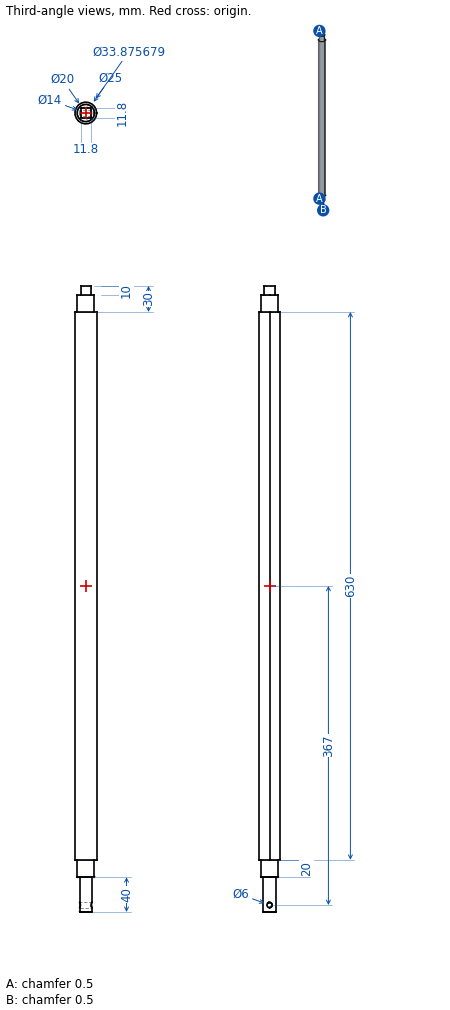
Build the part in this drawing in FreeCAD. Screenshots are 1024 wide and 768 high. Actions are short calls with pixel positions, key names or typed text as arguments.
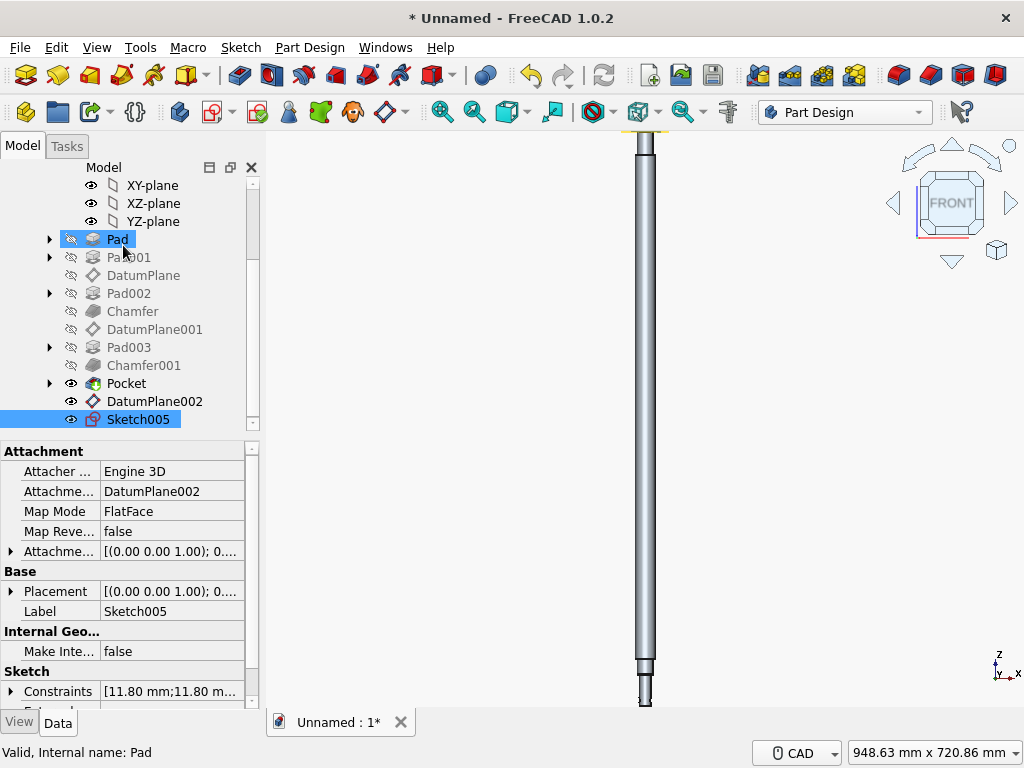
click(240, 76)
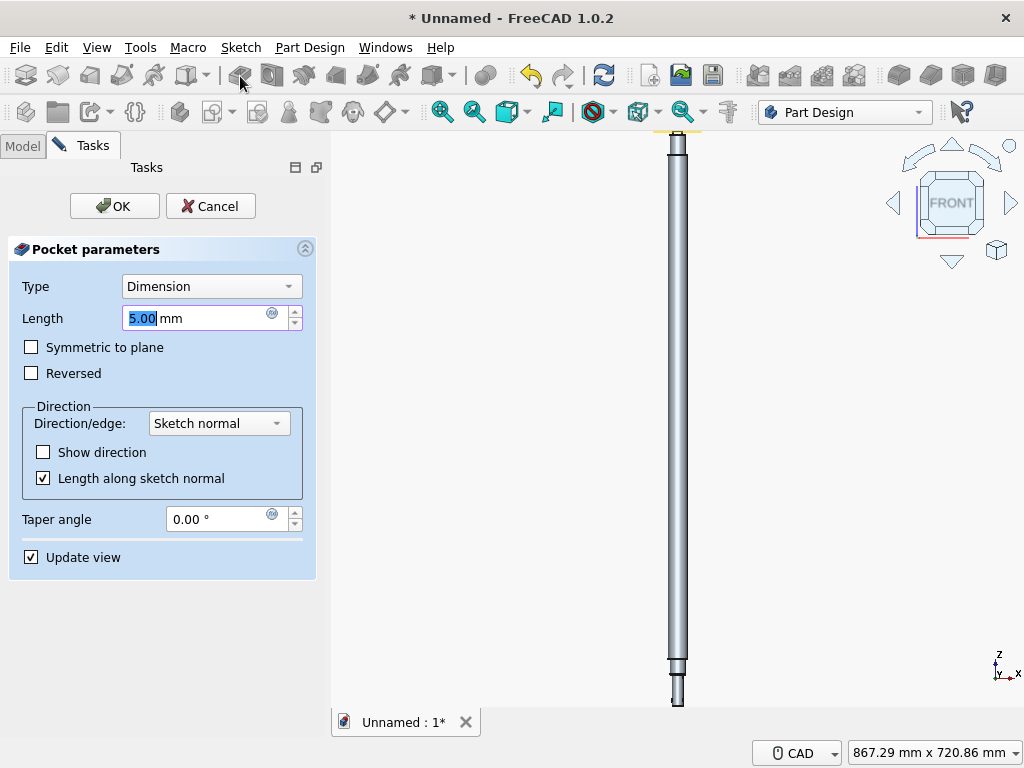
text(10)
key(Tab)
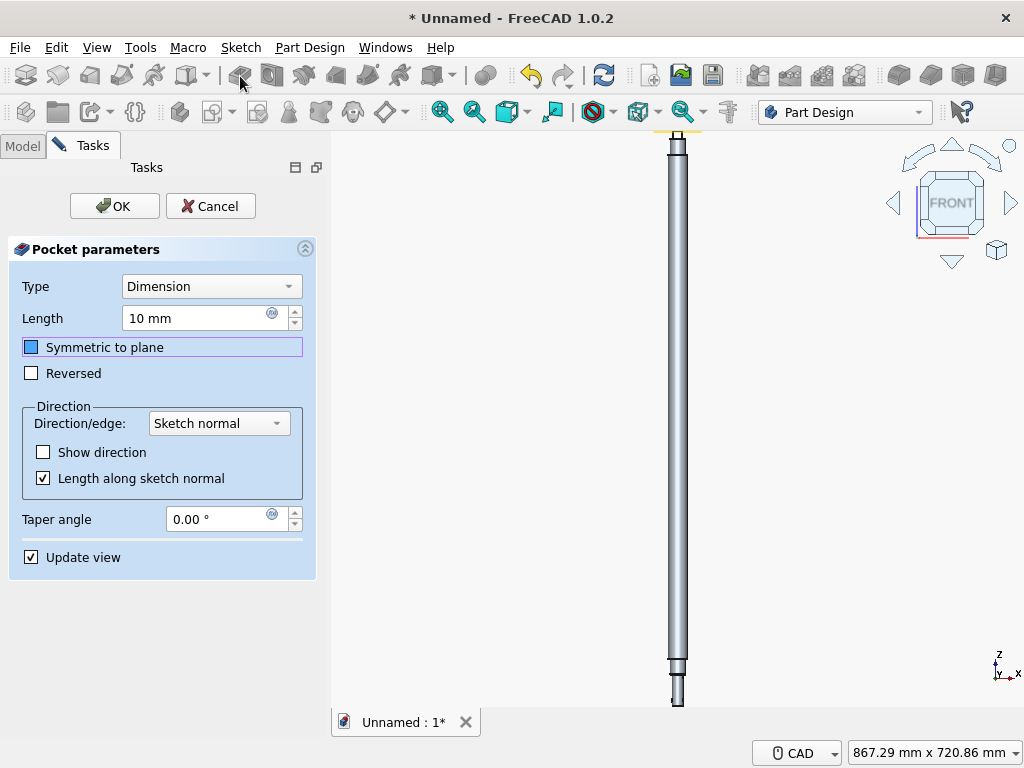
click(115, 206)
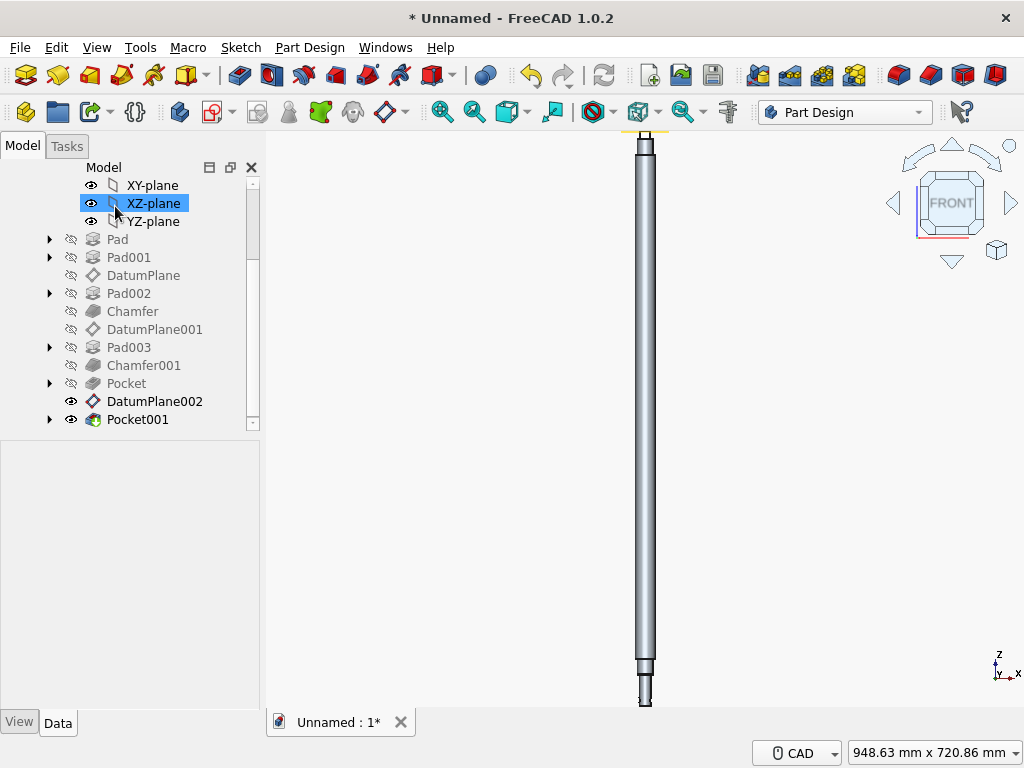
click(116, 401)
key(space)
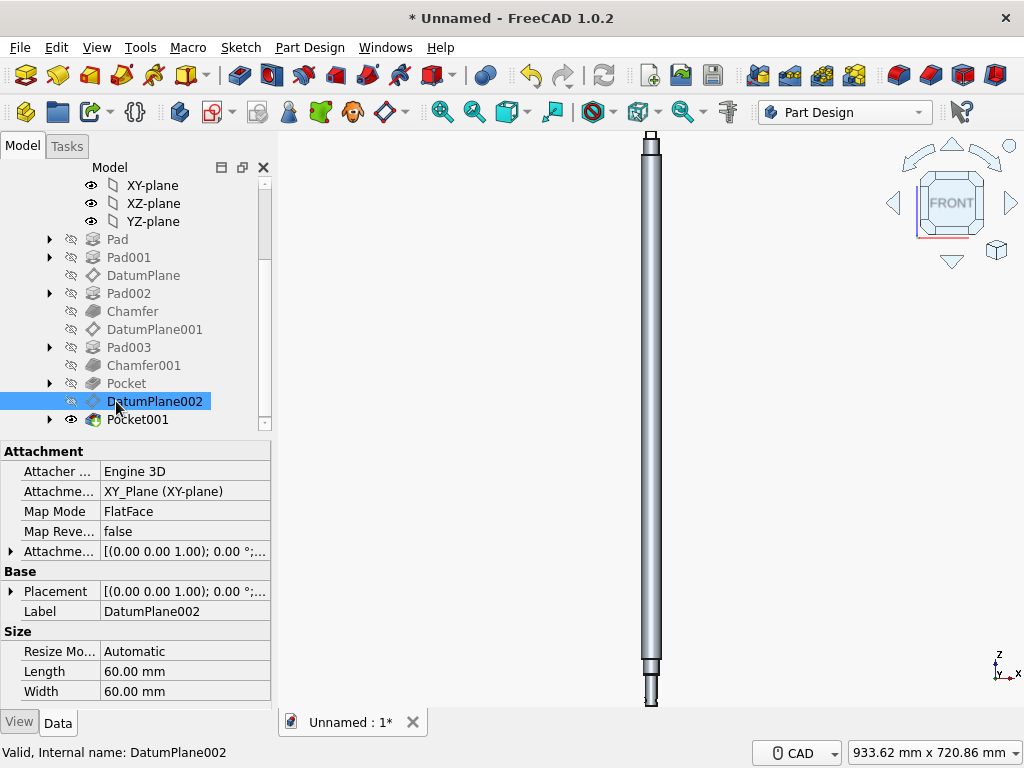
key(0)